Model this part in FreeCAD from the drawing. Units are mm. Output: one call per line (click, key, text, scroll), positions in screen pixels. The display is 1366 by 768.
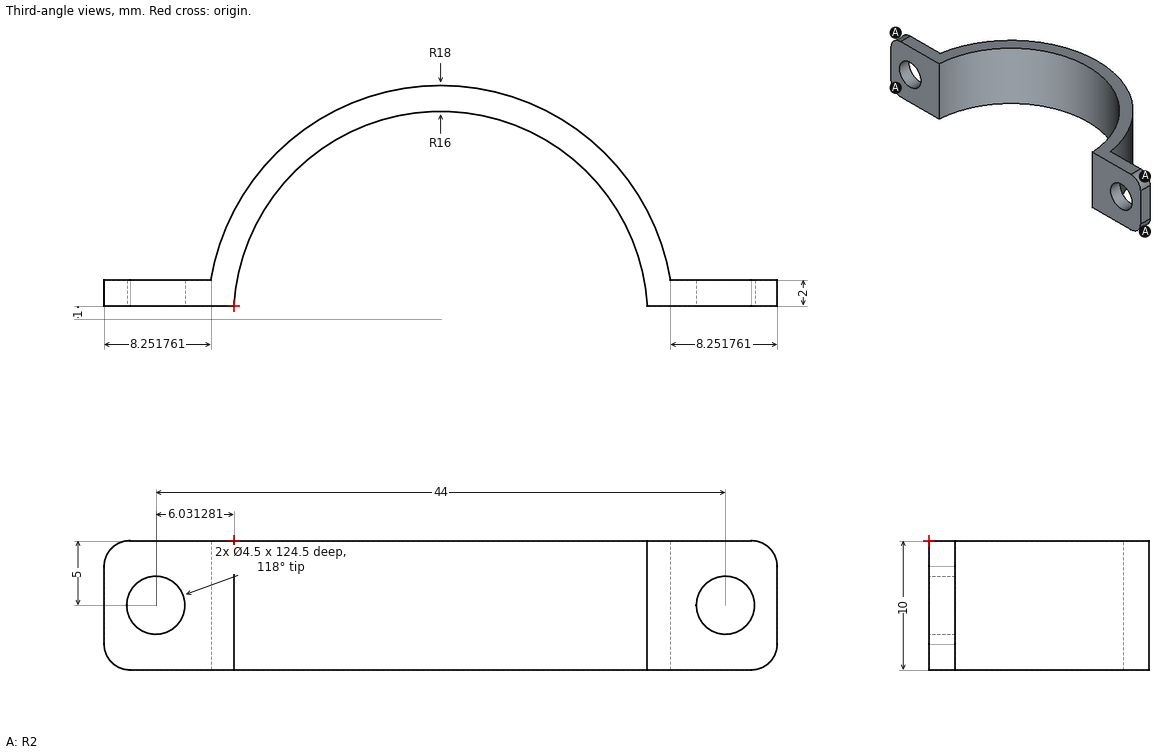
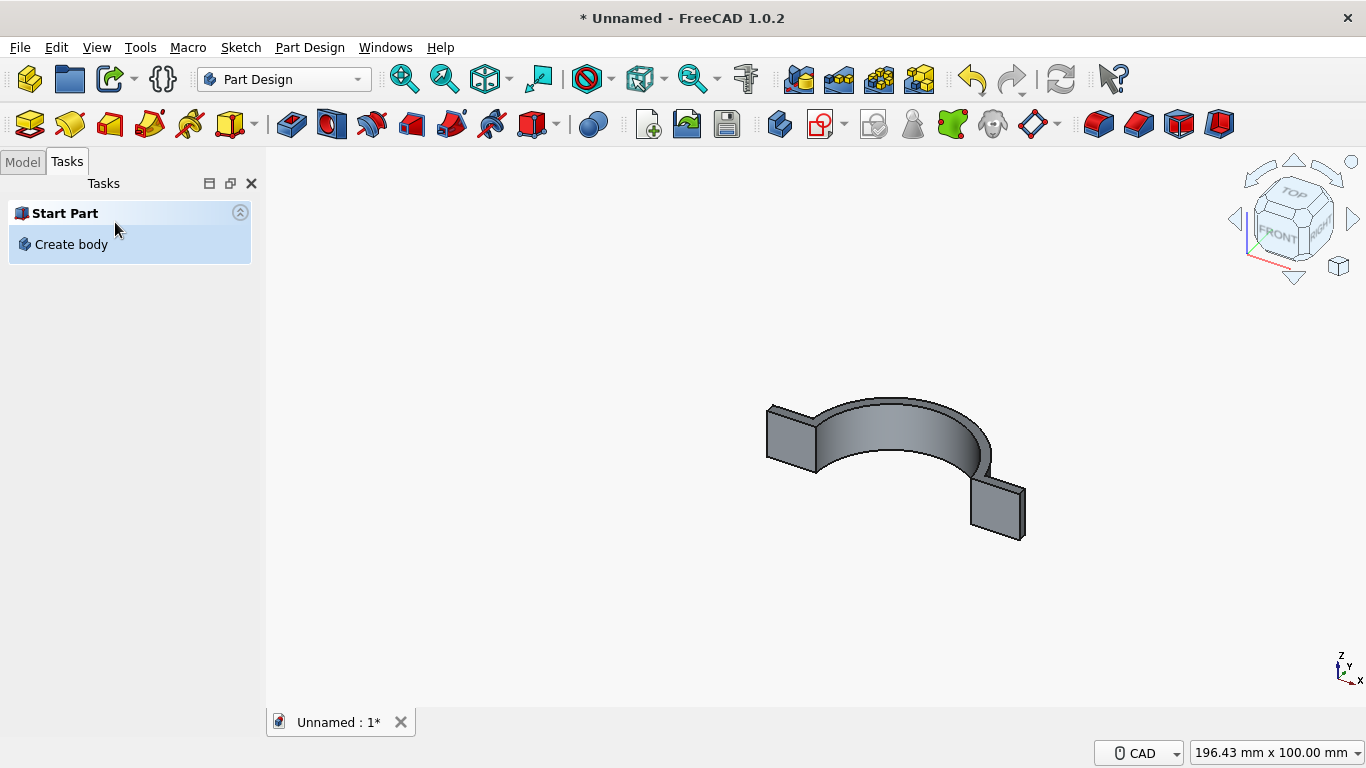
click(406, 80)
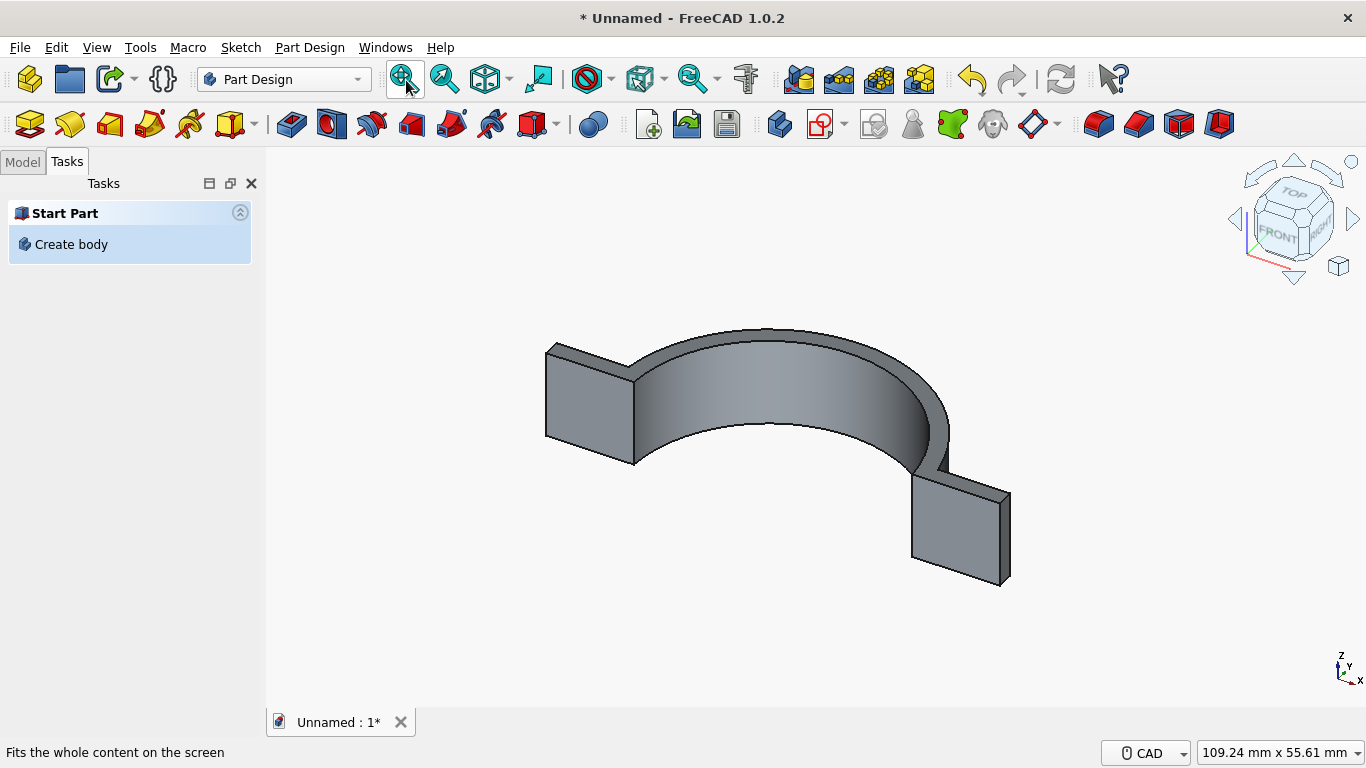
key(4)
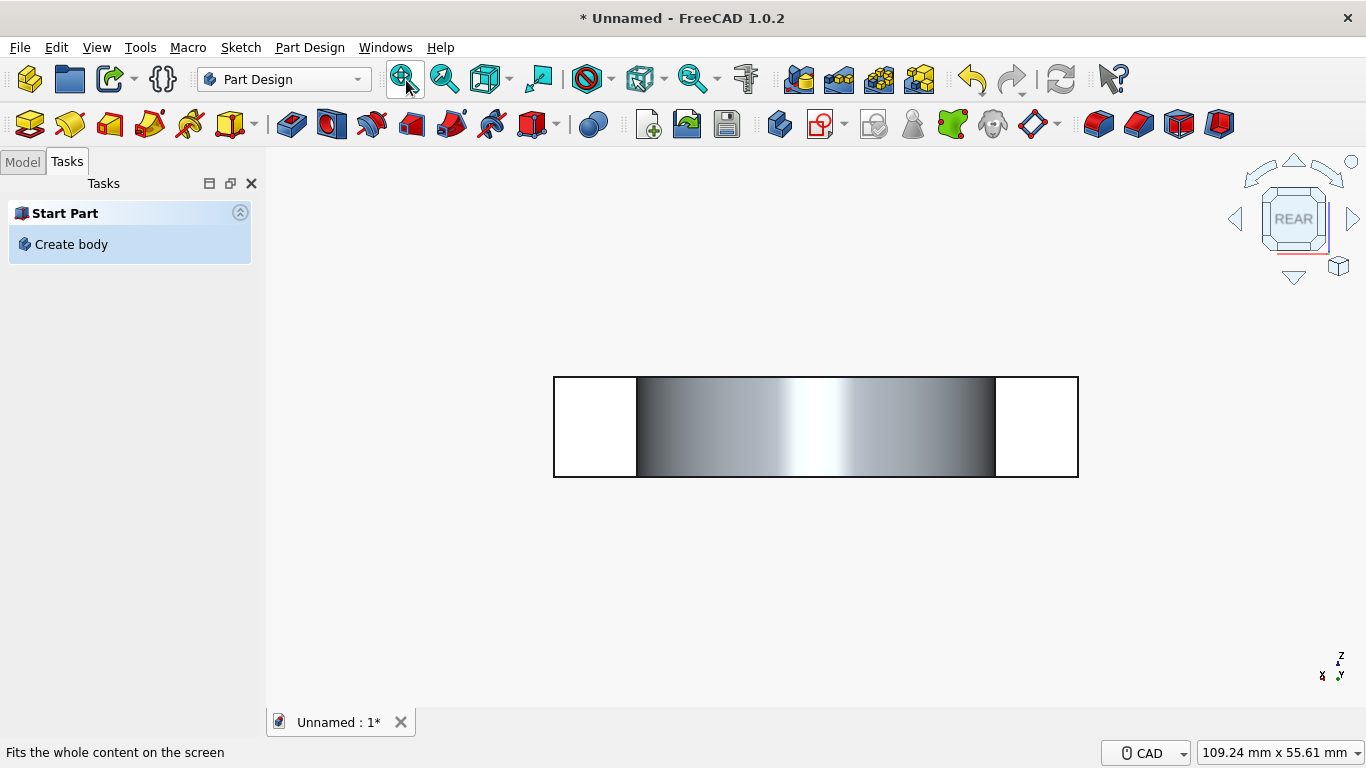
click(596, 426)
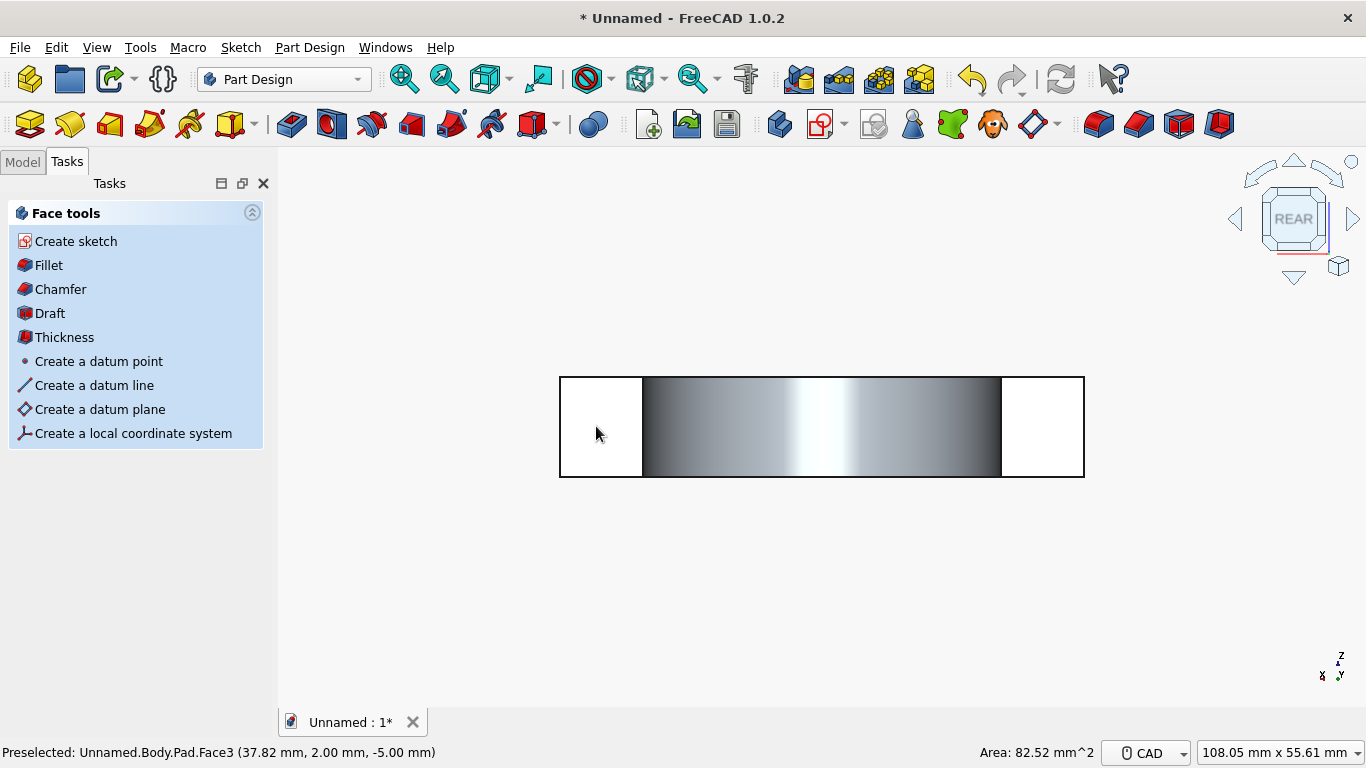
click(820, 124)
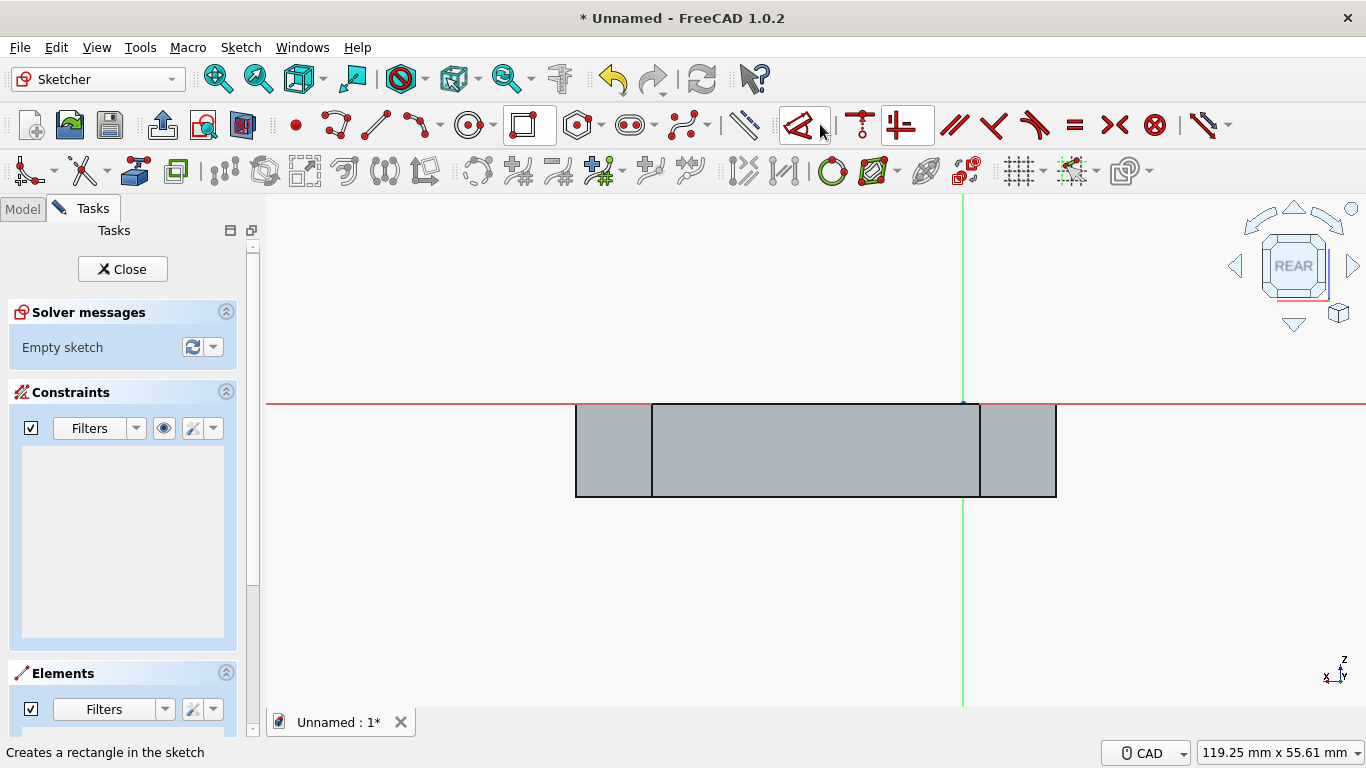
click(244, 126)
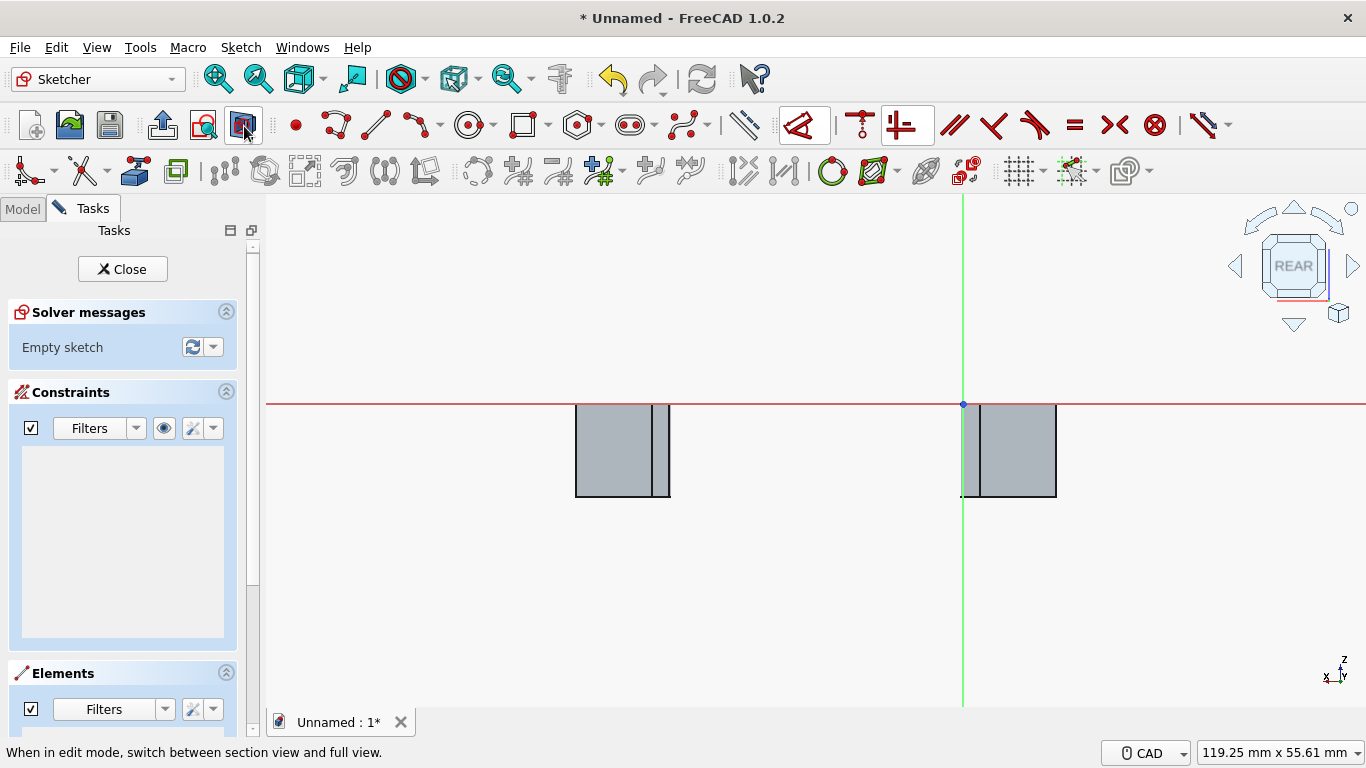
scroll(955, 412, up, 2)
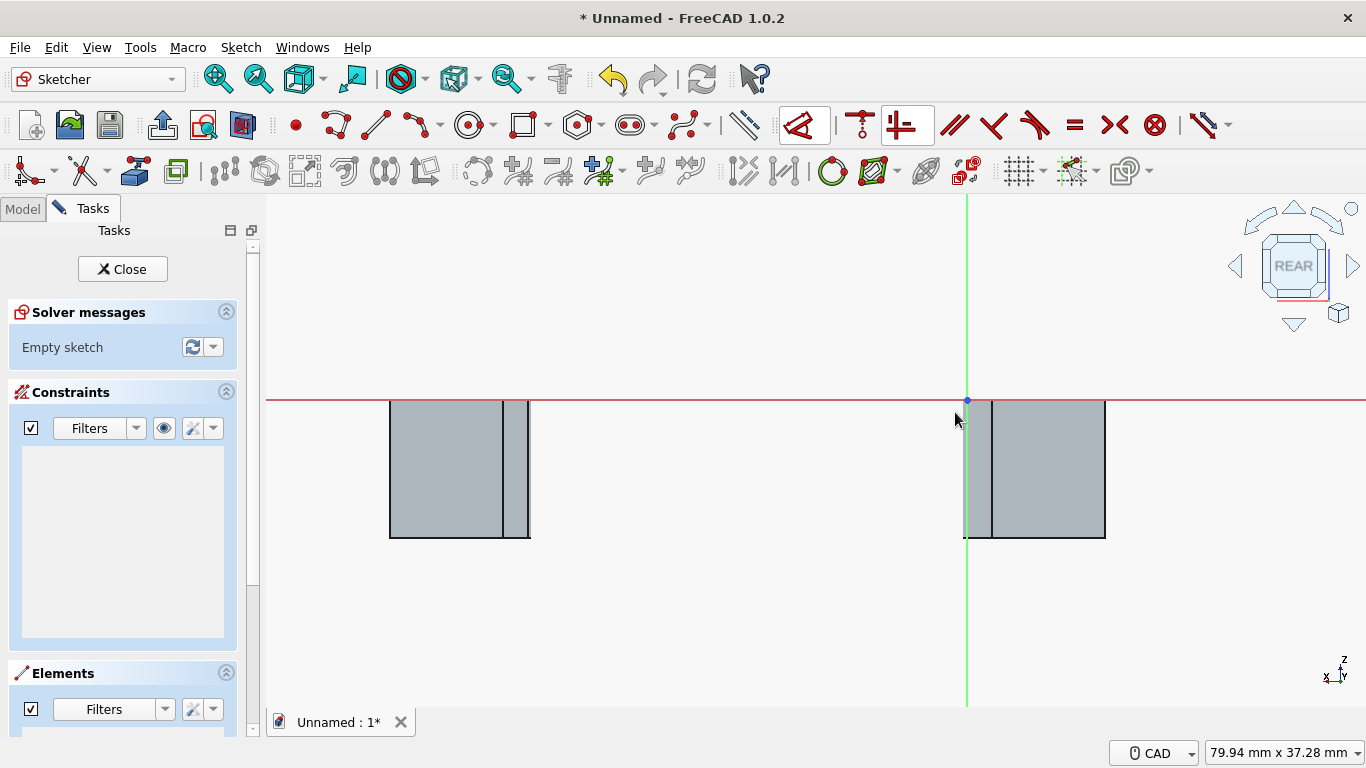
click(470, 126)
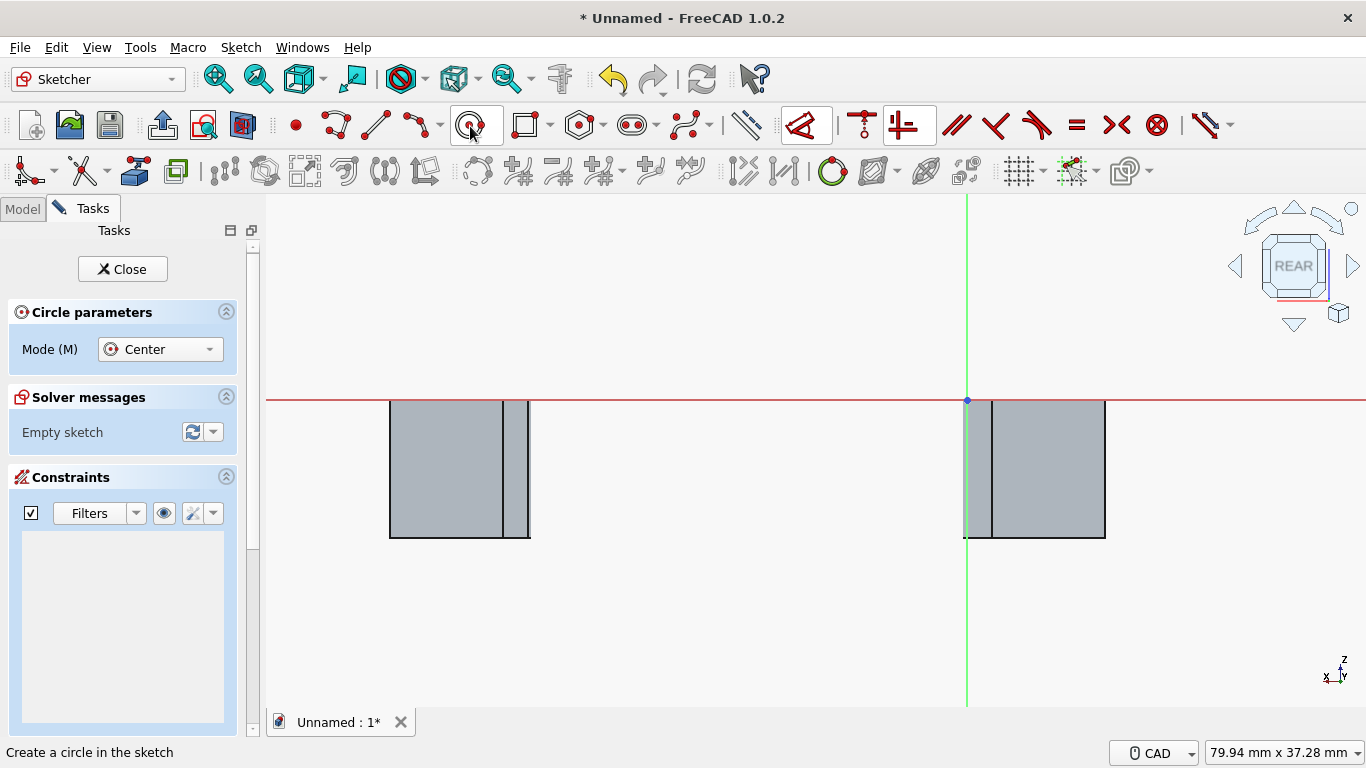
click(1050, 469)
move(1072, 447)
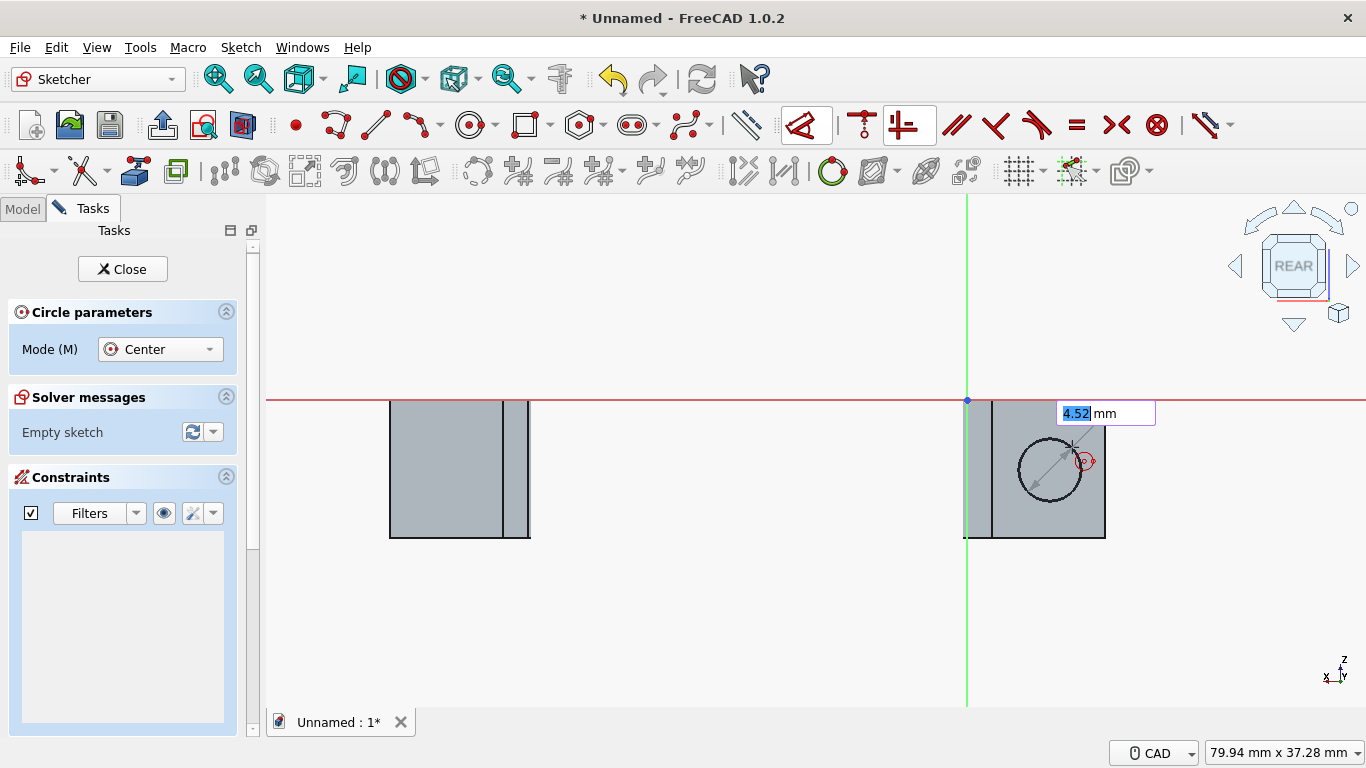
text(4.5)
key(Return)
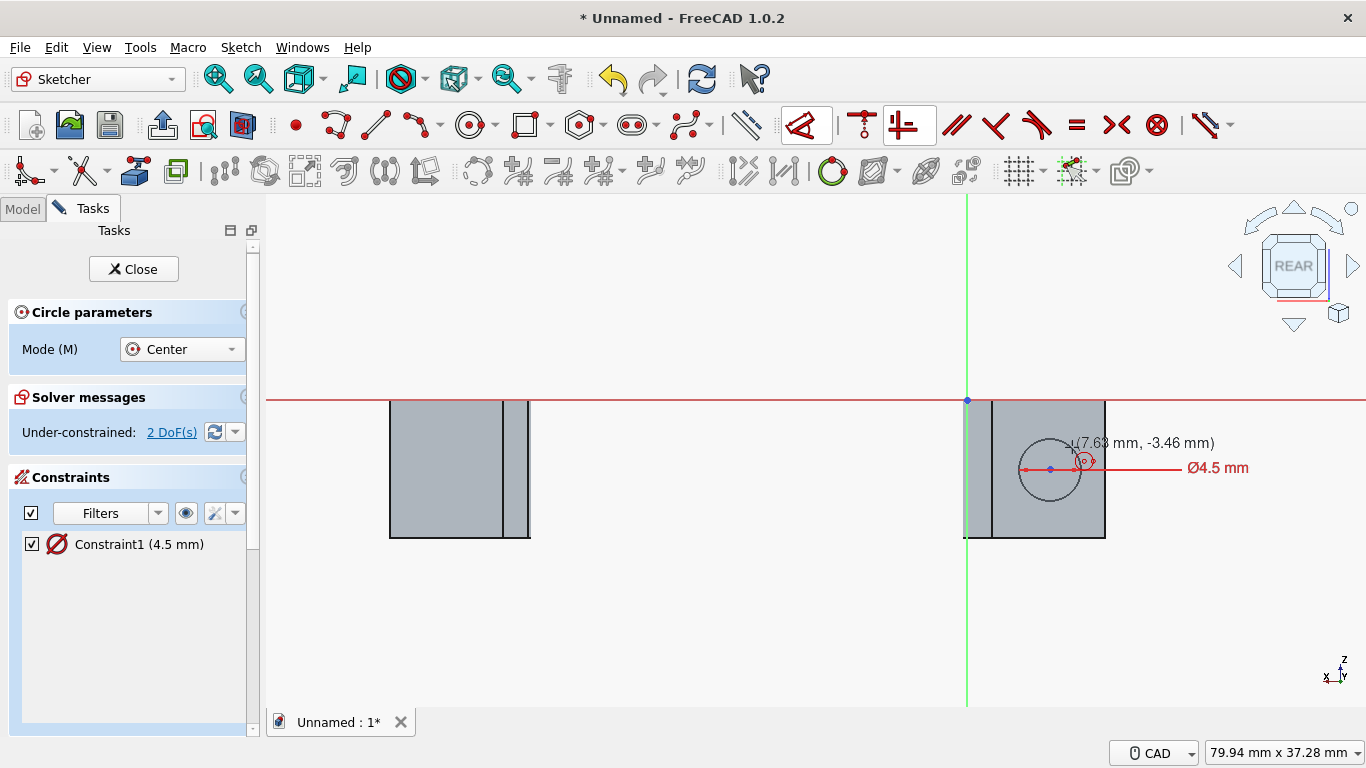
click(445, 469)
move(466, 447)